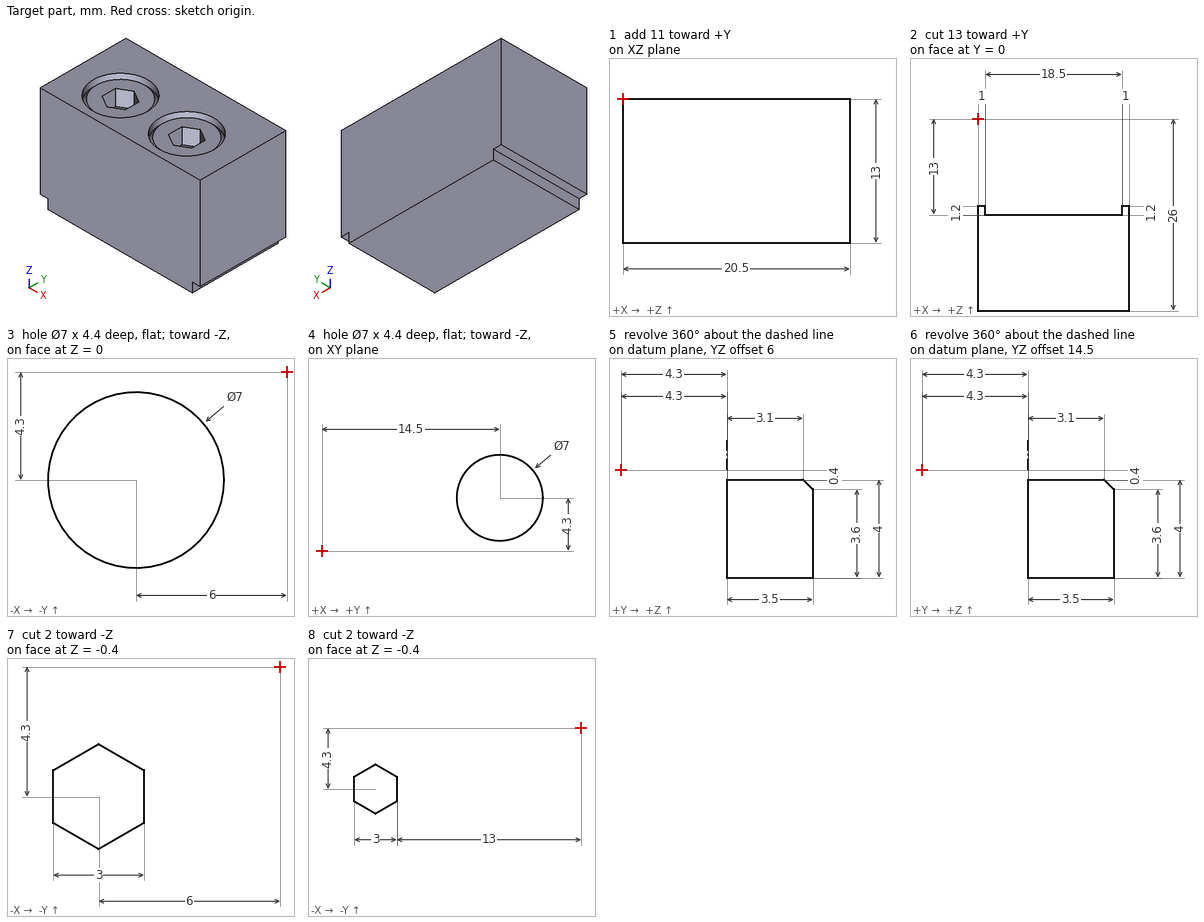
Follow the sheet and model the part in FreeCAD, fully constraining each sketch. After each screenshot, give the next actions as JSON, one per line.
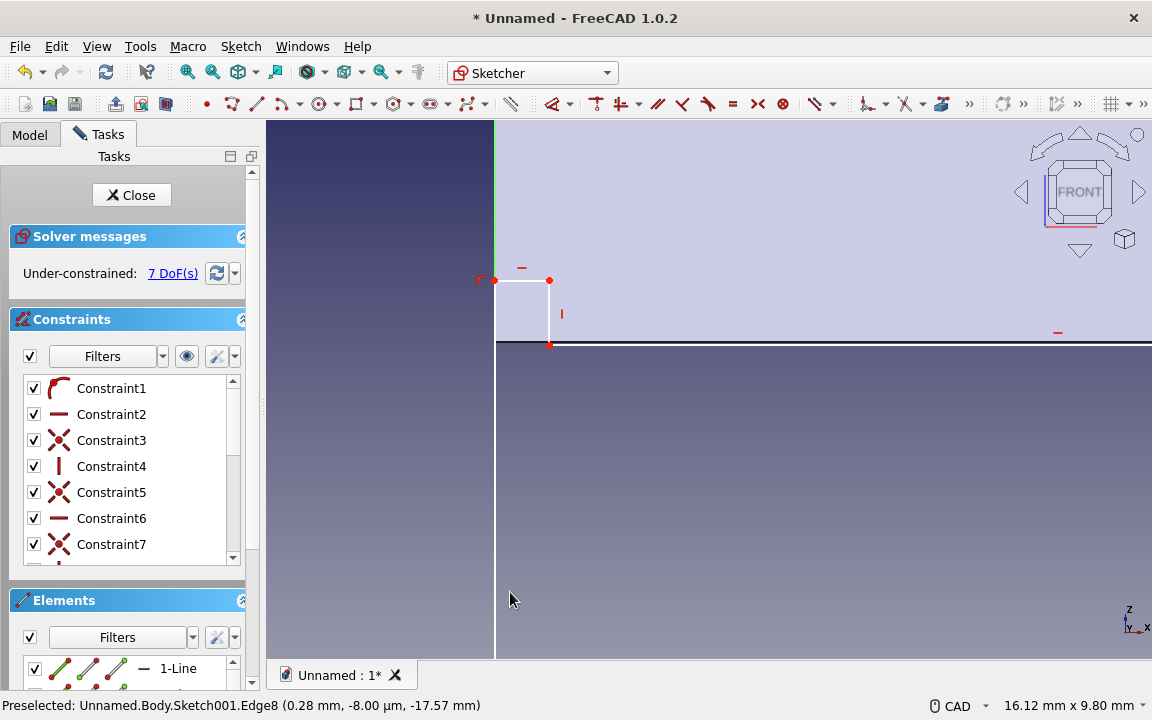
{"action": "left_click", "coordinate": [511, 281]}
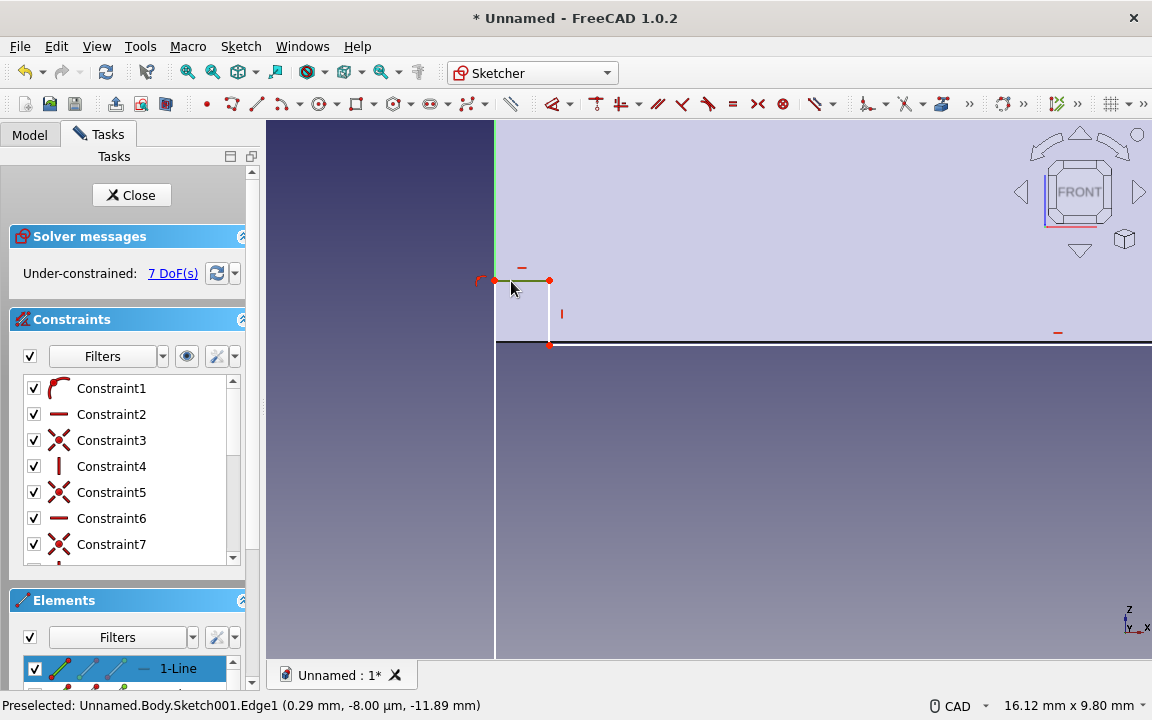
{"action": "key", "text": "l"}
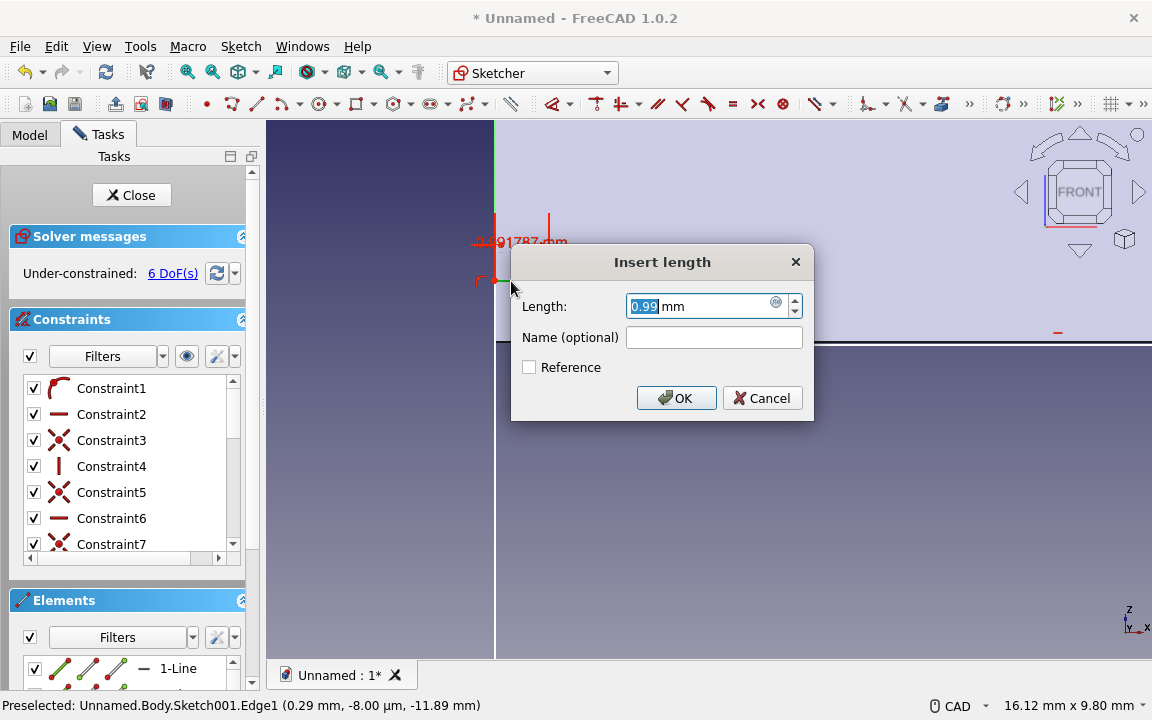
{"action": "type", "text": "1"}
{"action": "key", "text": "Return"}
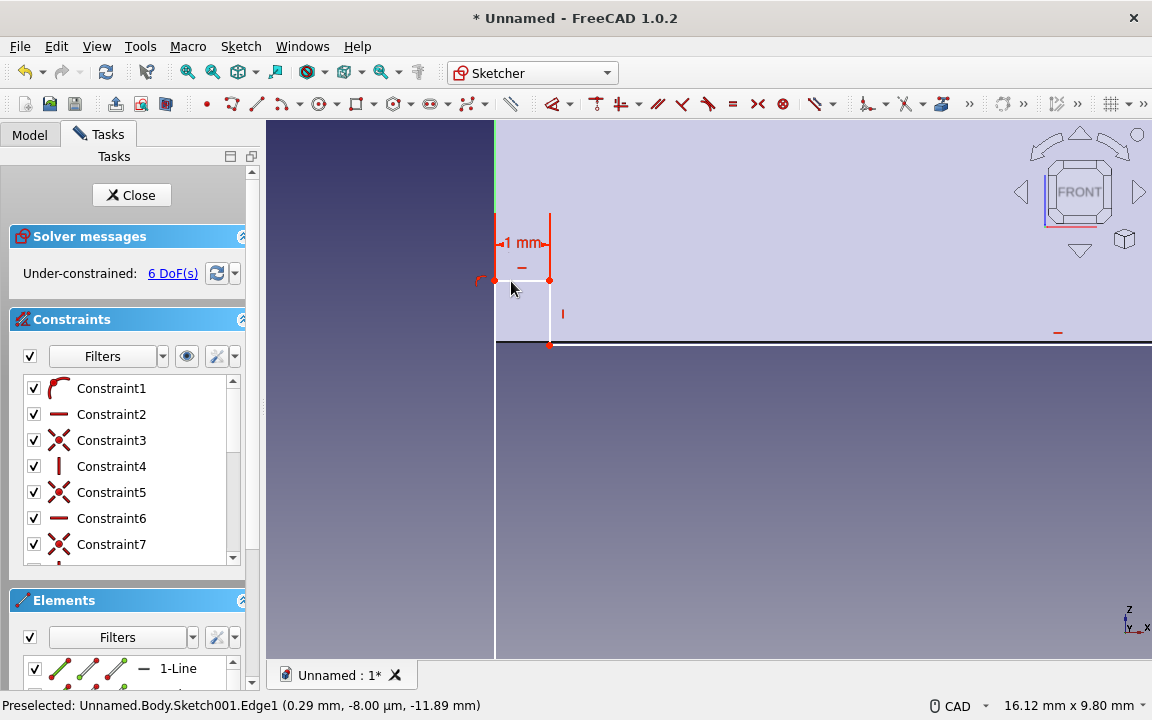
{"action": "scroll", "coordinate": [504, 405], "scroll_direction": "down", "scroll_amount": 7}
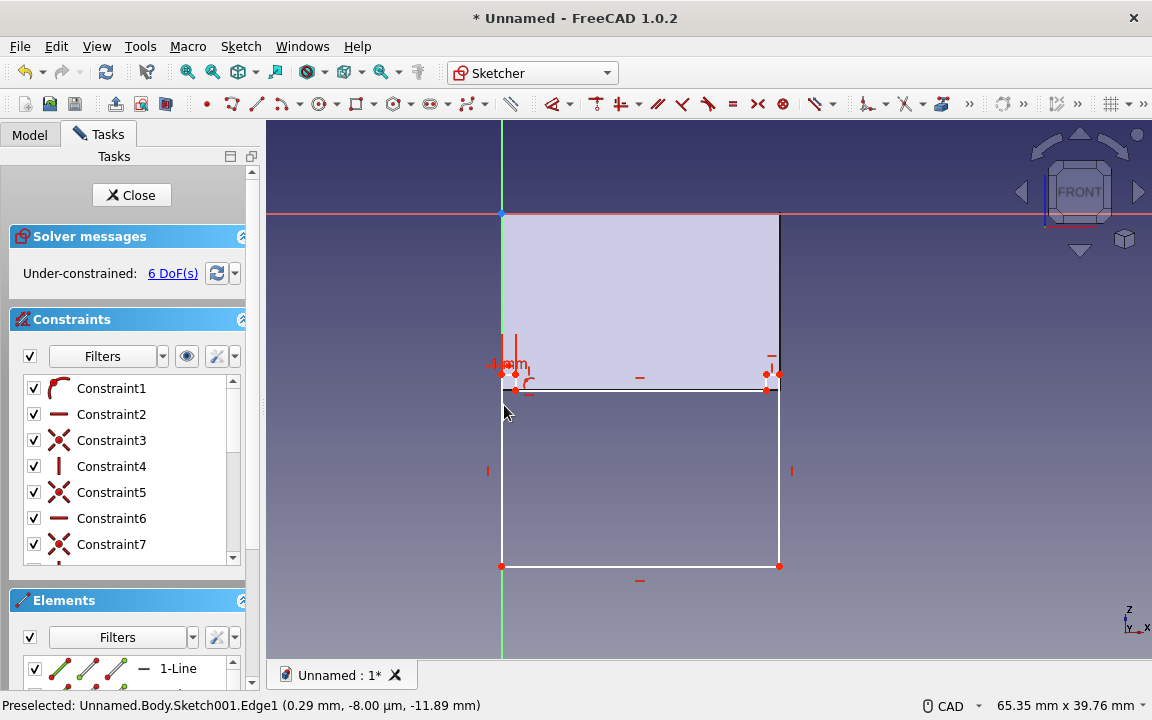
{"action": "scroll", "coordinate": [770, 375], "scroll_direction": "up", "scroll_amount": 7}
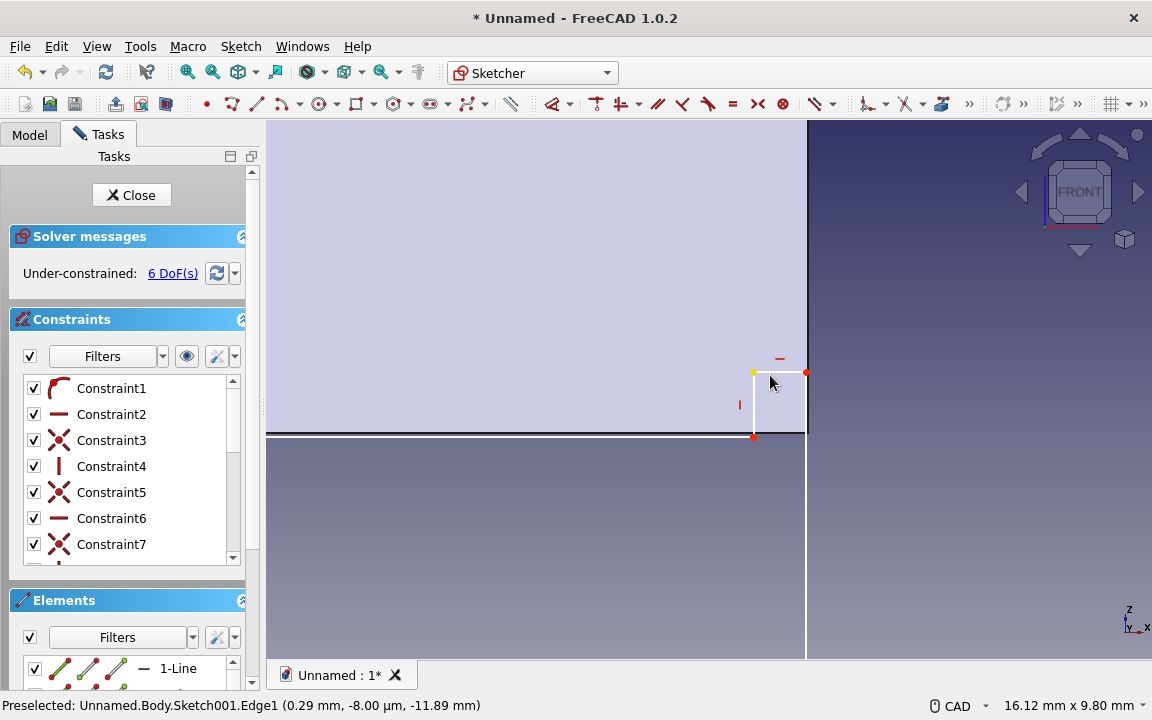
{"action": "left_click", "coordinate": [770, 372]}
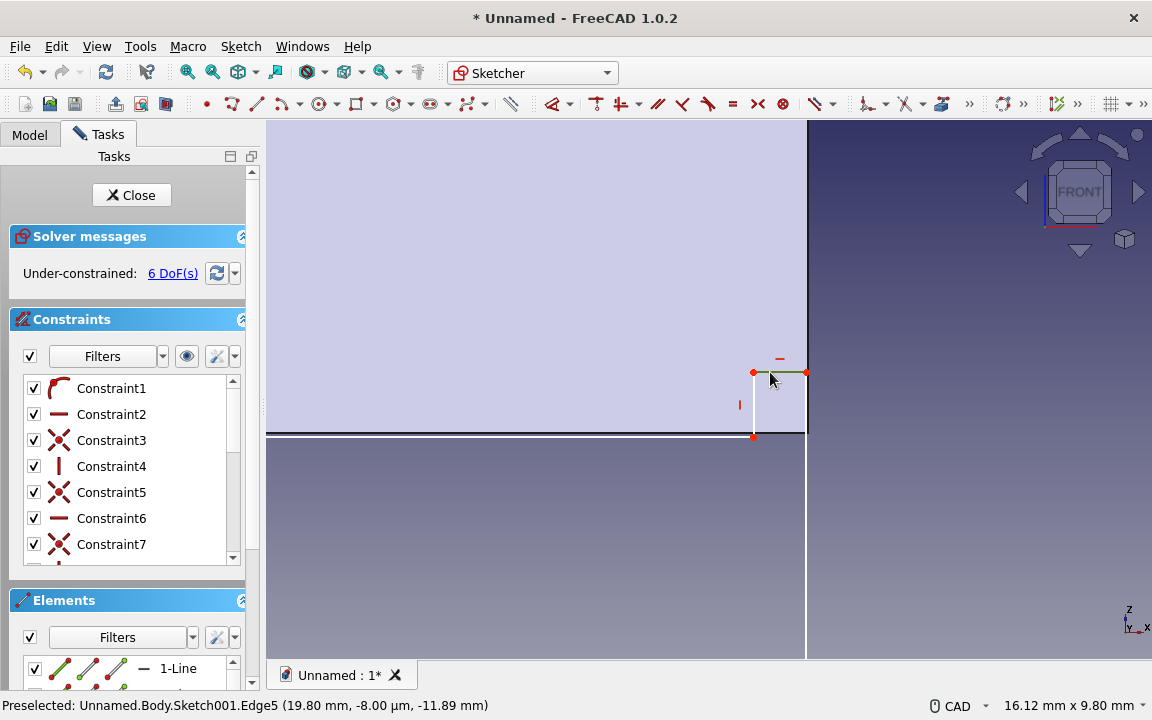
{"action": "left_click", "coordinate": [570, 104]}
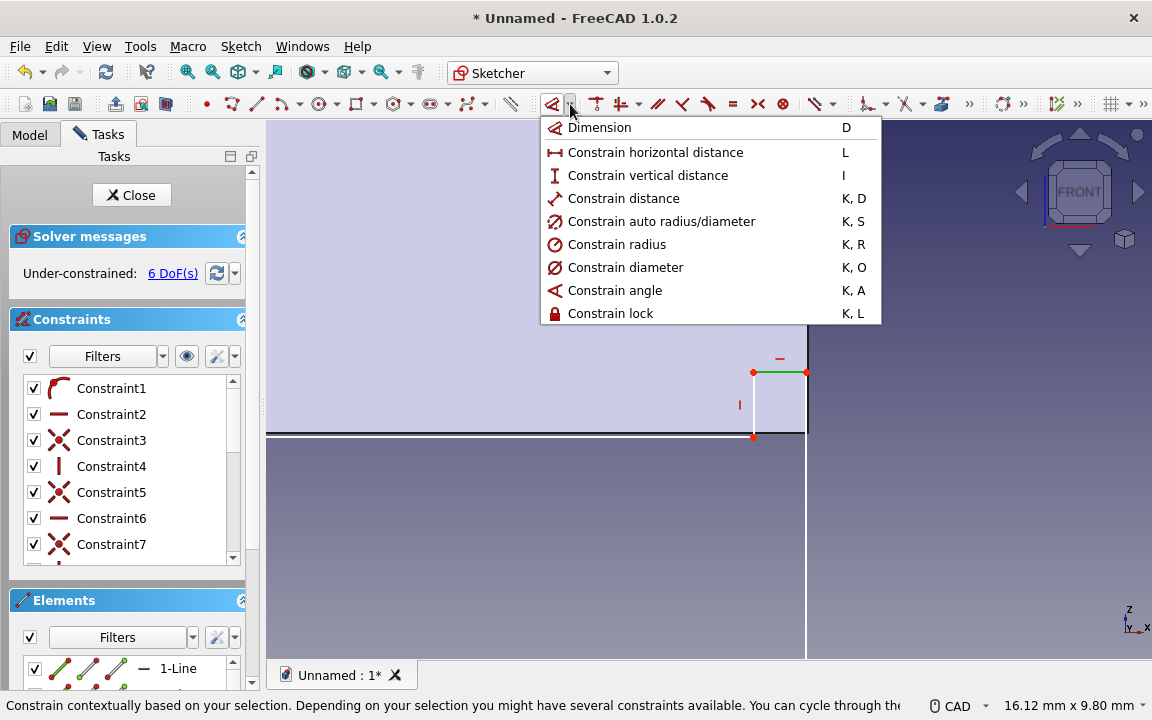
{"action": "left_click", "coordinate": [711, 152]}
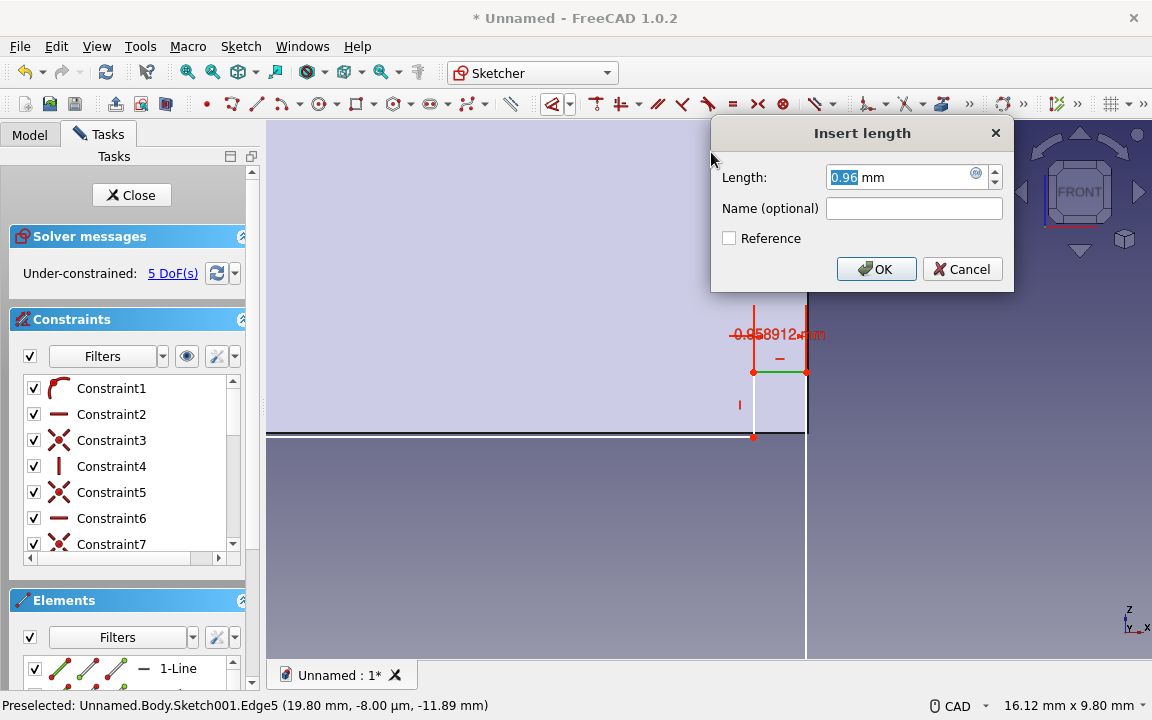
{"action": "type", "text": "1"}
{"action": "key", "text": "Return"}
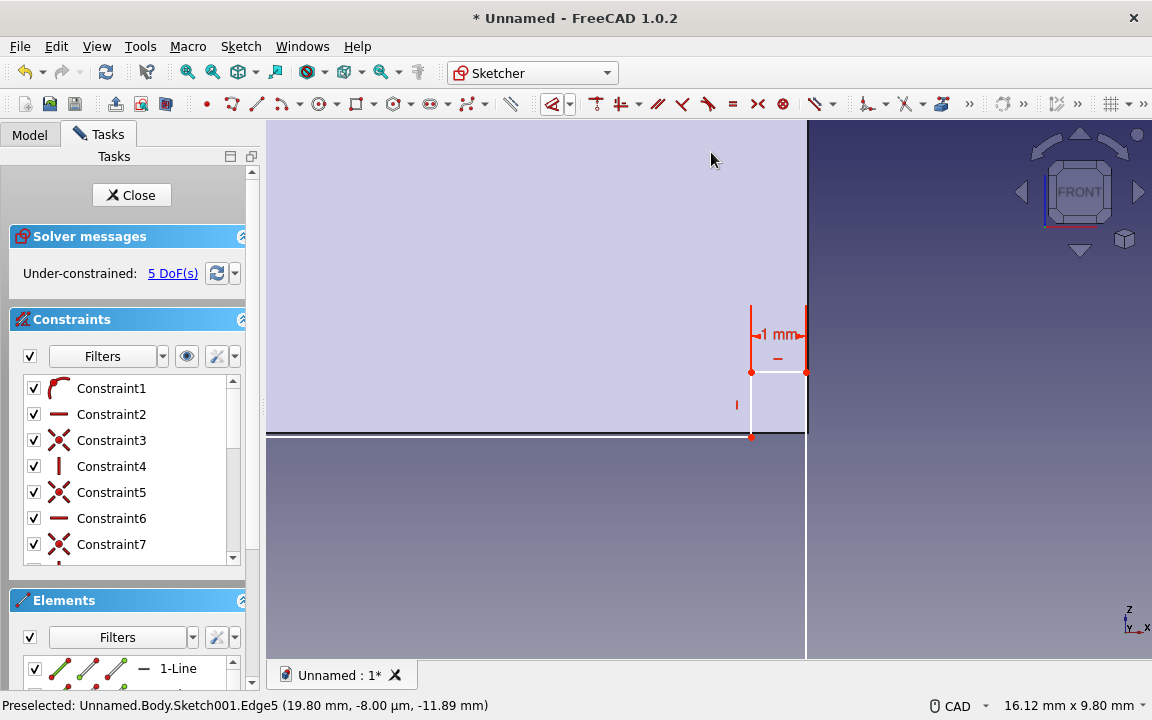
{"action": "scroll", "coordinate": [770, 375], "scroll_direction": "down", "scroll_amount": 7}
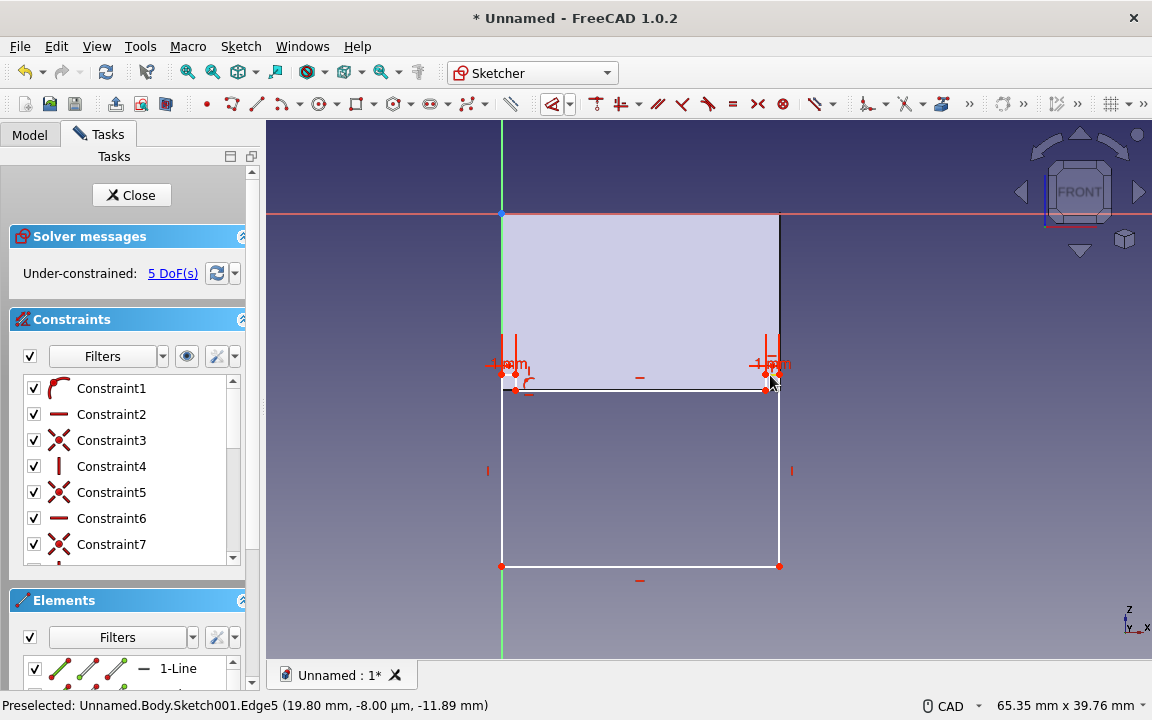
{"action": "scroll", "coordinate": [516, 380], "scroll_direction": "up", "scroll_amount": 6}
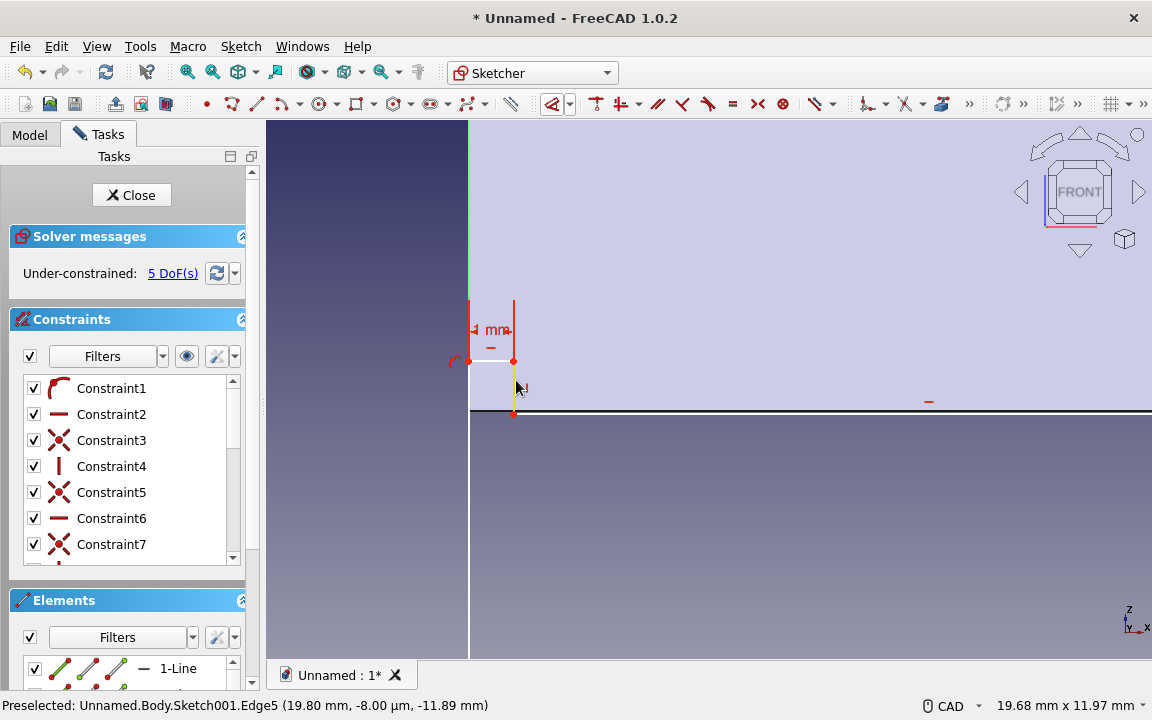
{"action": "left_click", "coordinate": [514, 377]}